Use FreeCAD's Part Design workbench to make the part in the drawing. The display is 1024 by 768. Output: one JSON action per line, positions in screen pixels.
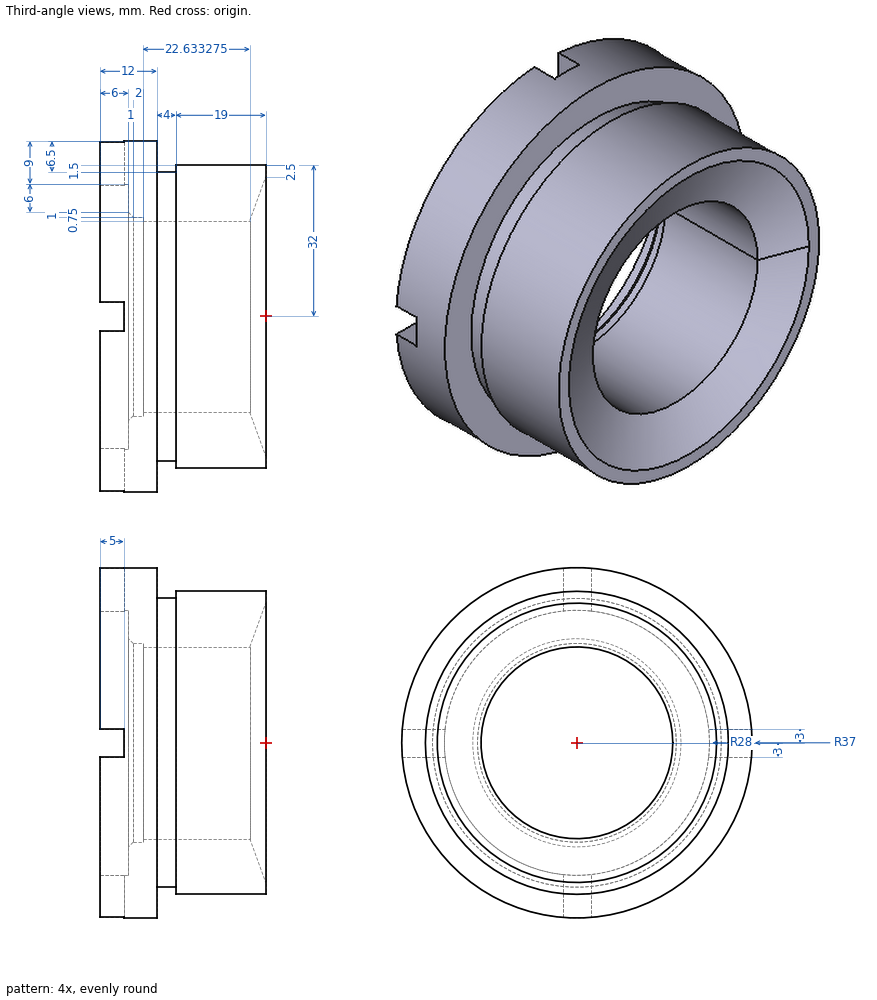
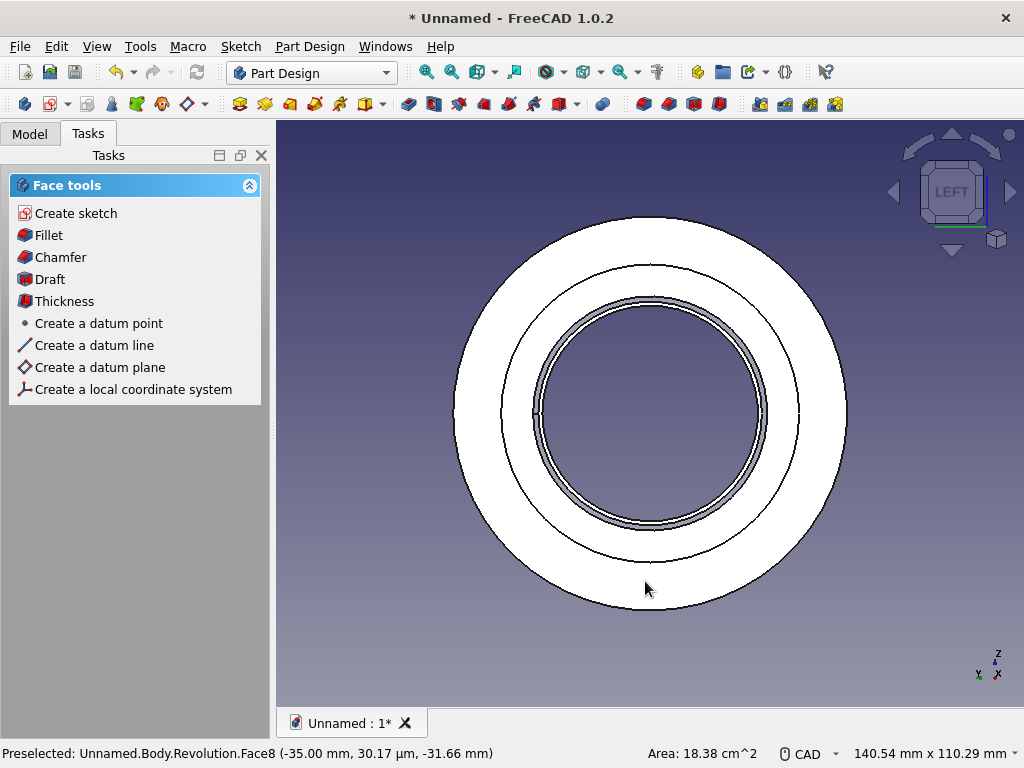
{"action": "left_click", "coordinate": [50, 104]}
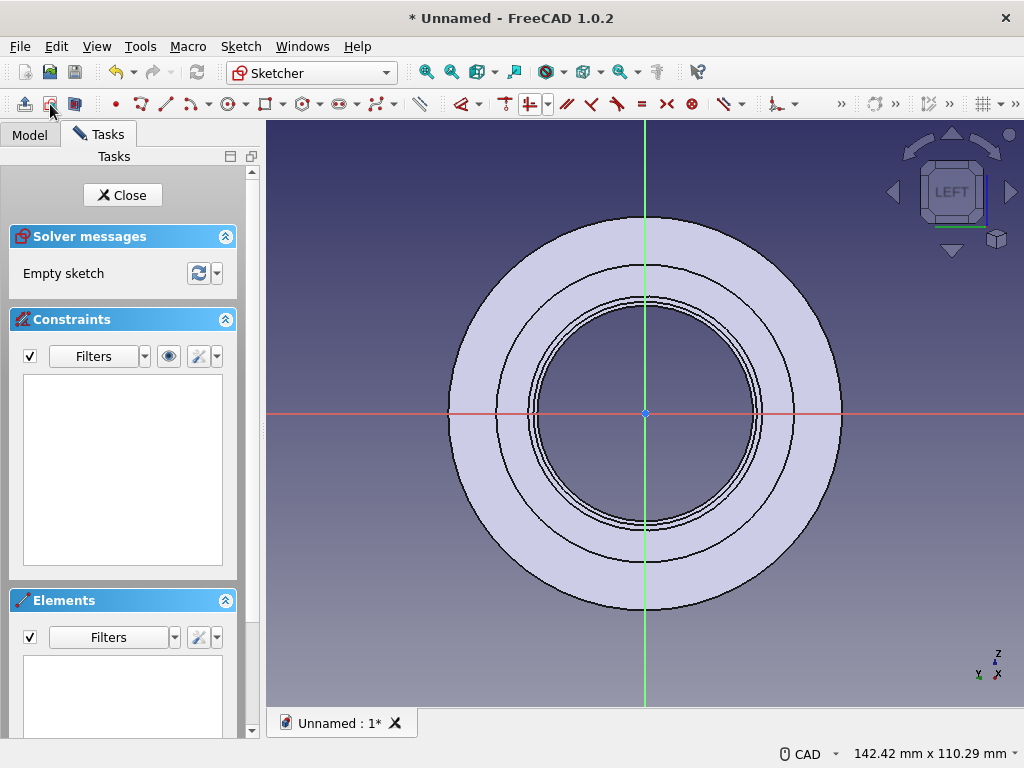
{"action": "scroll", "coordinate": [460, 414], "scroll_direction": "up", "scroll_amount": 11}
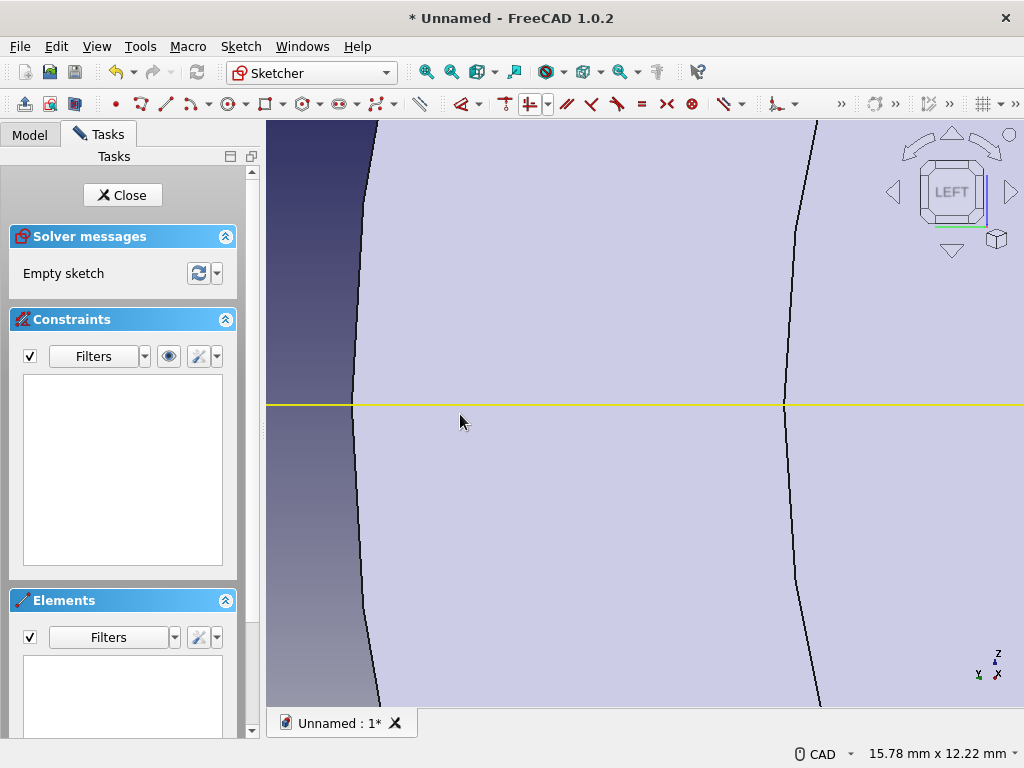
{"action": "left_click", "coordinate": [166, 104]}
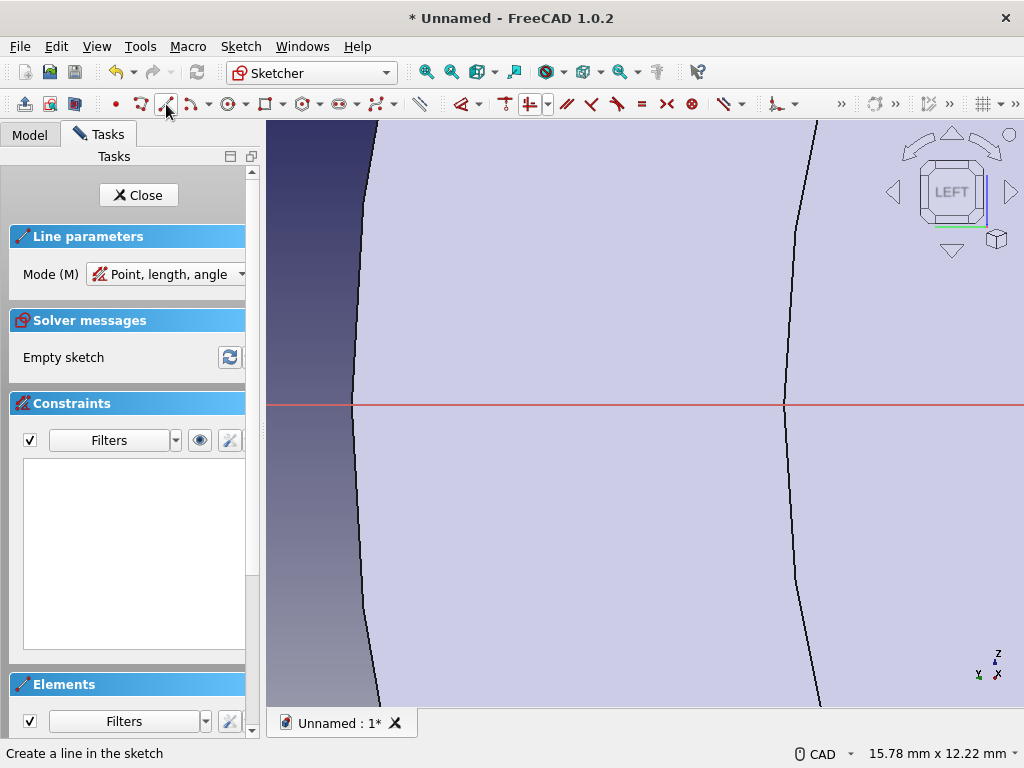
{"action": "left_click", "coordinate": [358, 550]}
{"action": "left_click", "coordinate": [792, 550]}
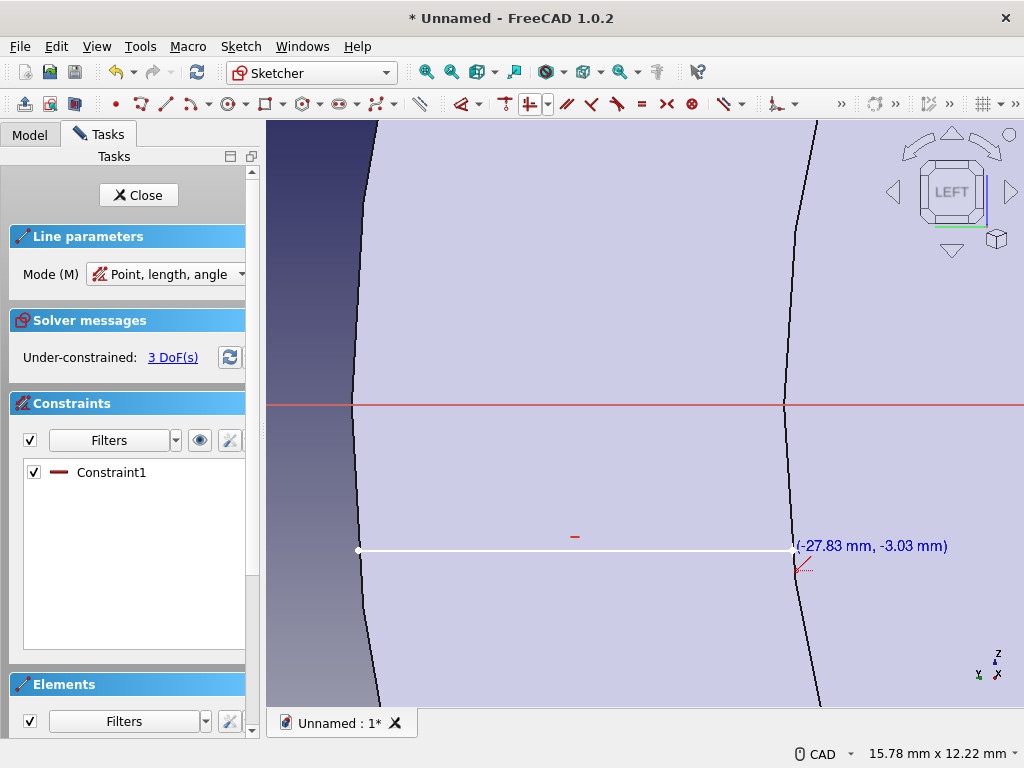
{"action": "left_click", "coordinate": [792, 261]}
{"action": "left_click", "coordinate": [358, 261]}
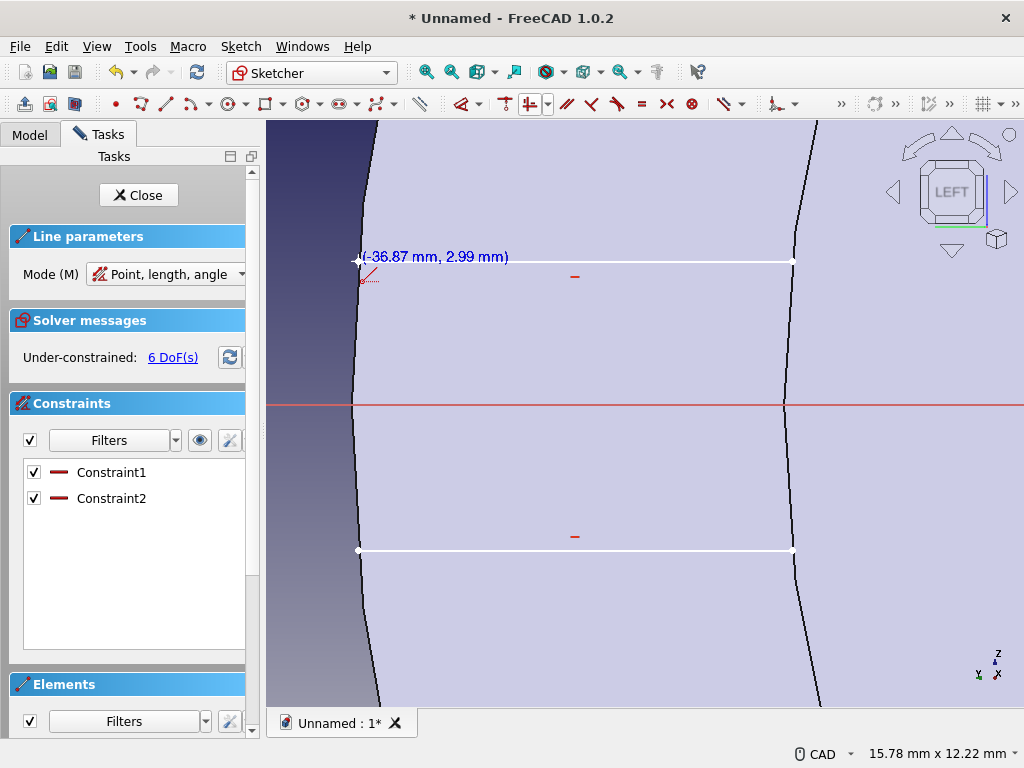
{"action": "left_click", "coordinate": [208, 104]}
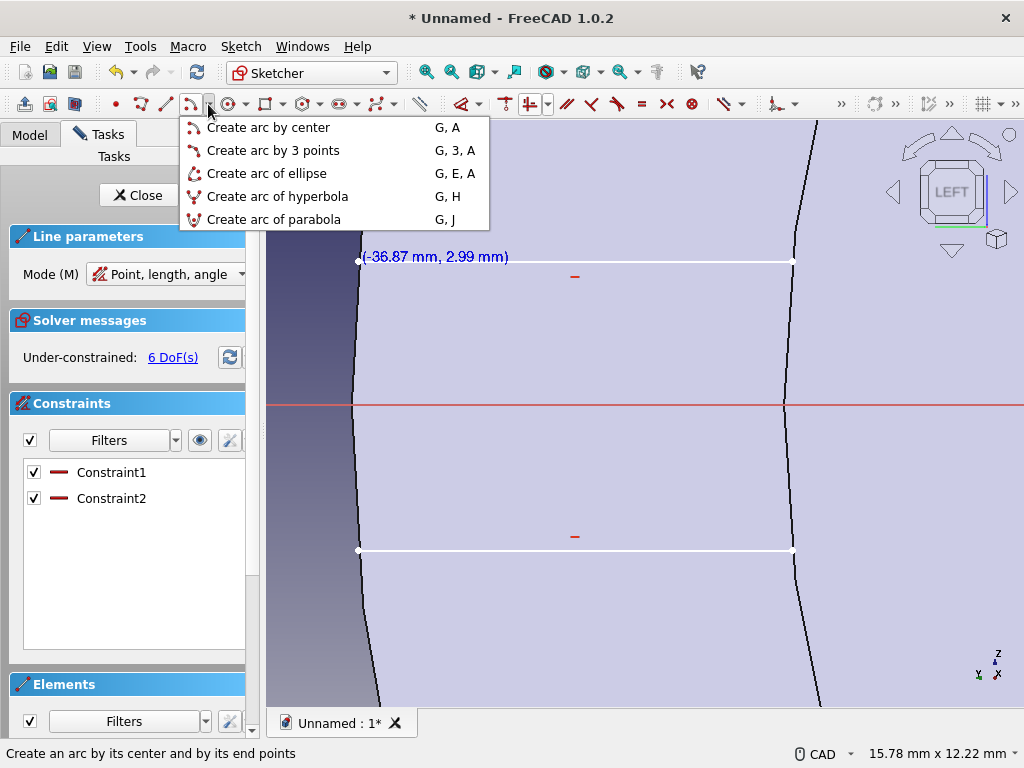
{"action": "left_click", "coordinate": [334, 150]}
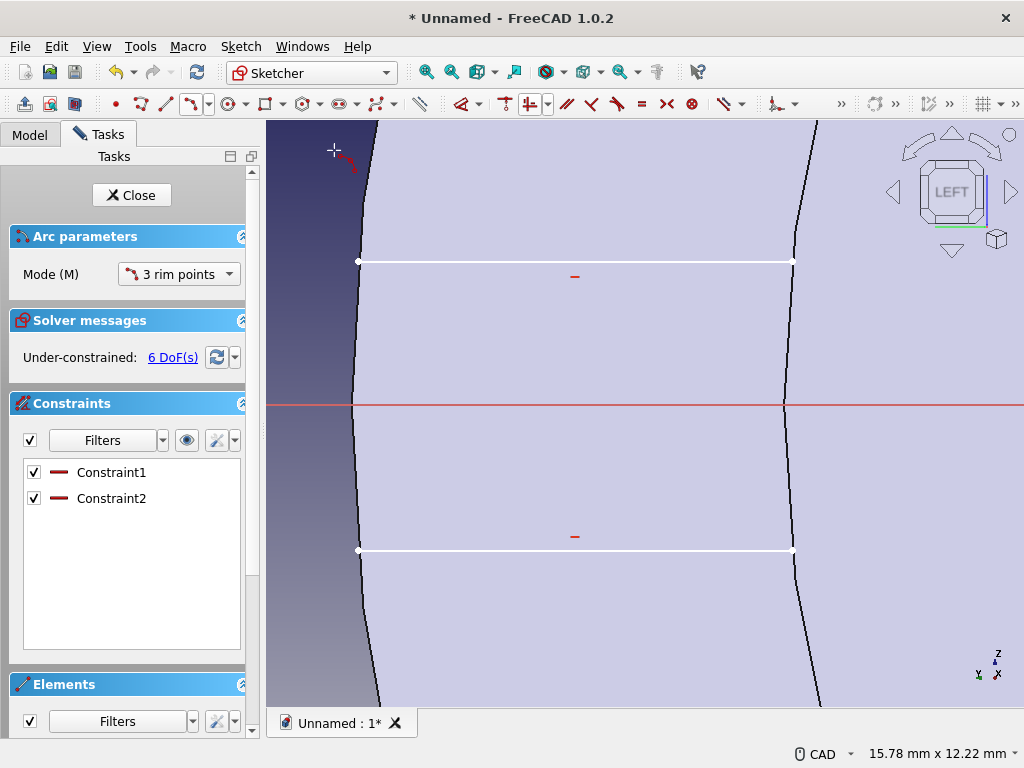
{"action": "left_click", "coordinate": [792, 551]}
{"action": "left_click", "coordinate": [792, 262]}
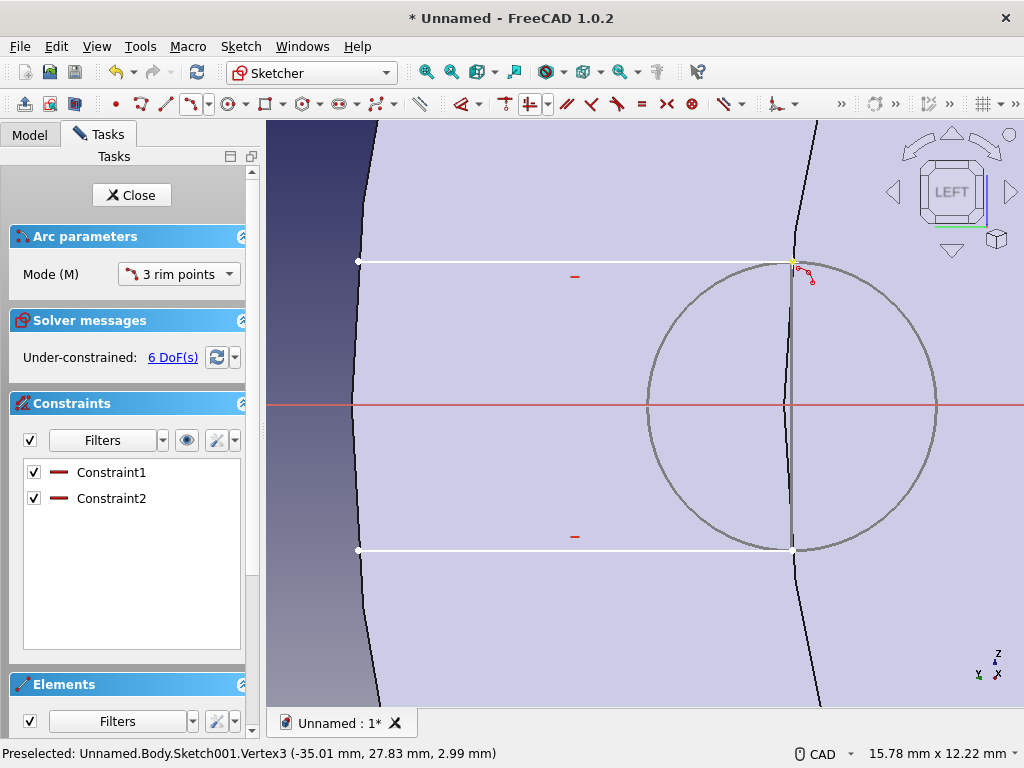
{"action": "scroll", "coordinate": [784, 377], "scroll_direction": "up", "scroll_amount": 4}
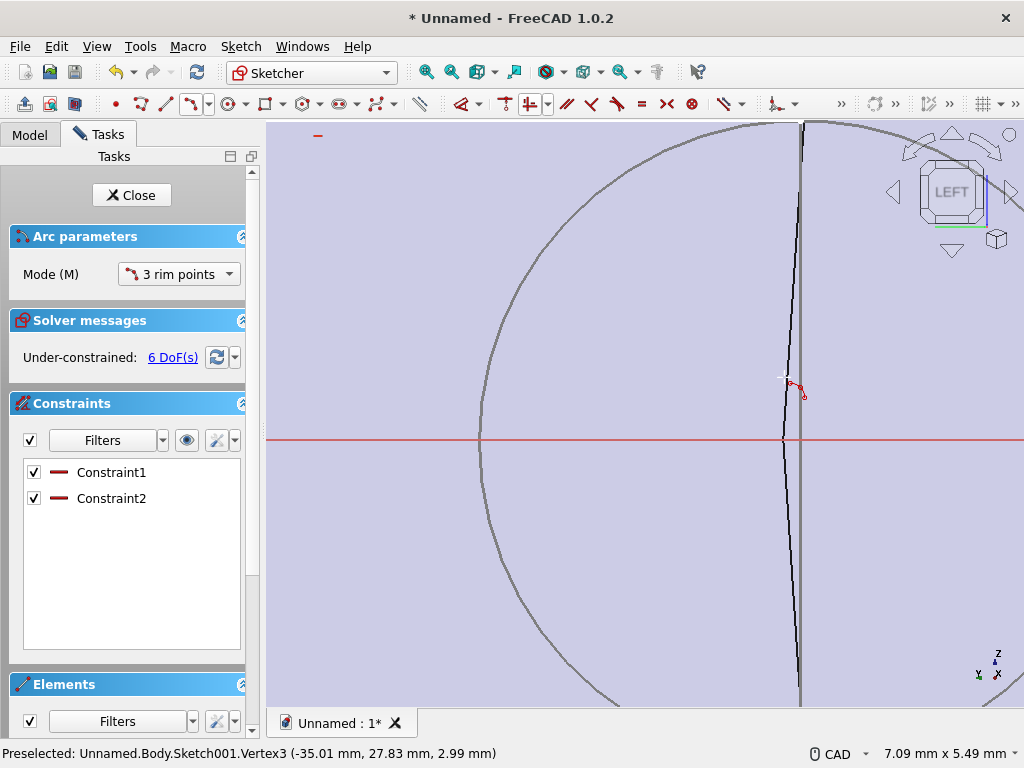
{"action": "left_click", "coordinate": [784, 376]}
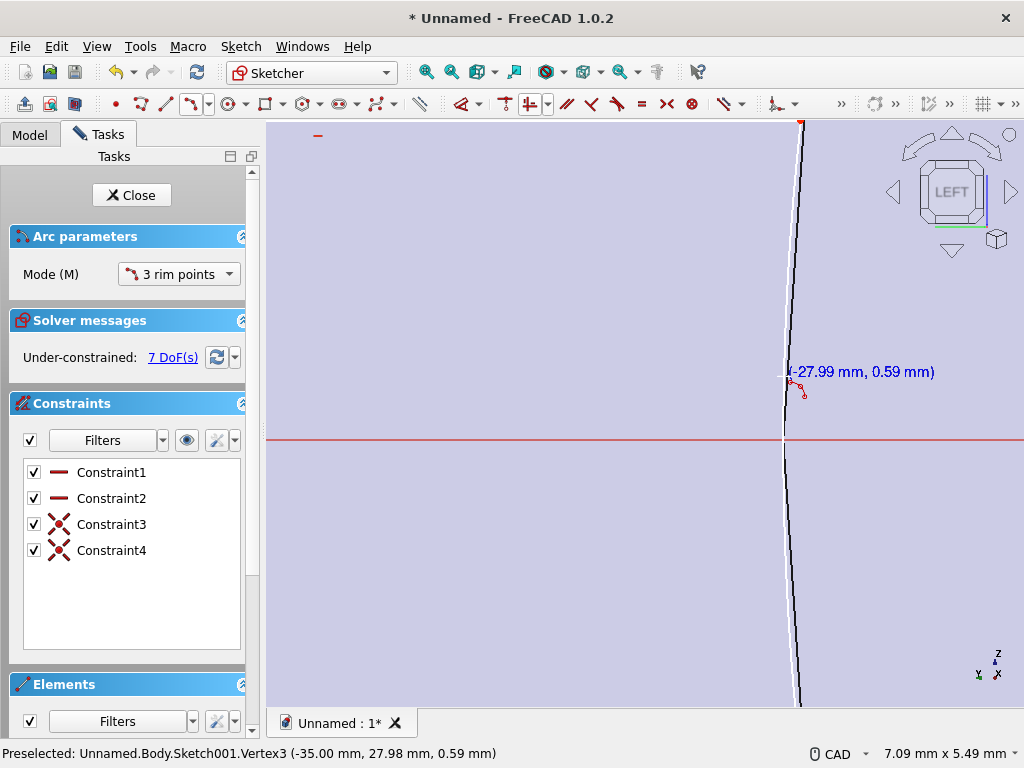
{"action": "scroll", "coordinate": [793, 392], "scroll_direction": "down", "scroll_amount": 4}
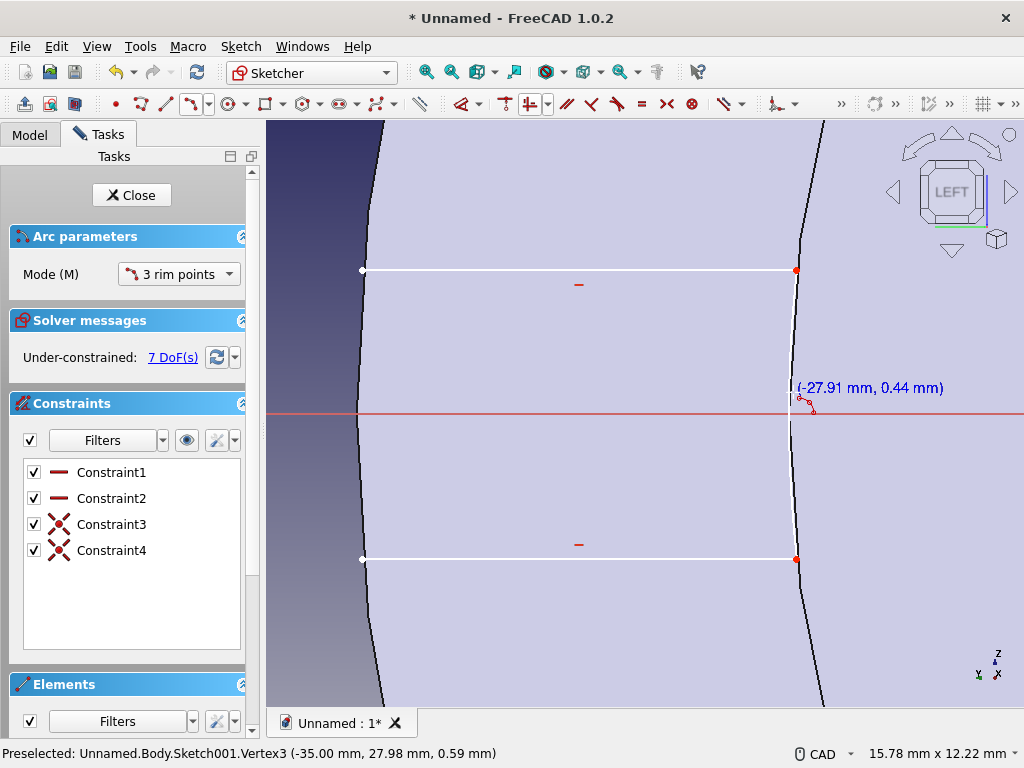
{"action": "left_click", "coordinate": [363, 270]}
{"action": "left_click", "coordinate": [363, 559]}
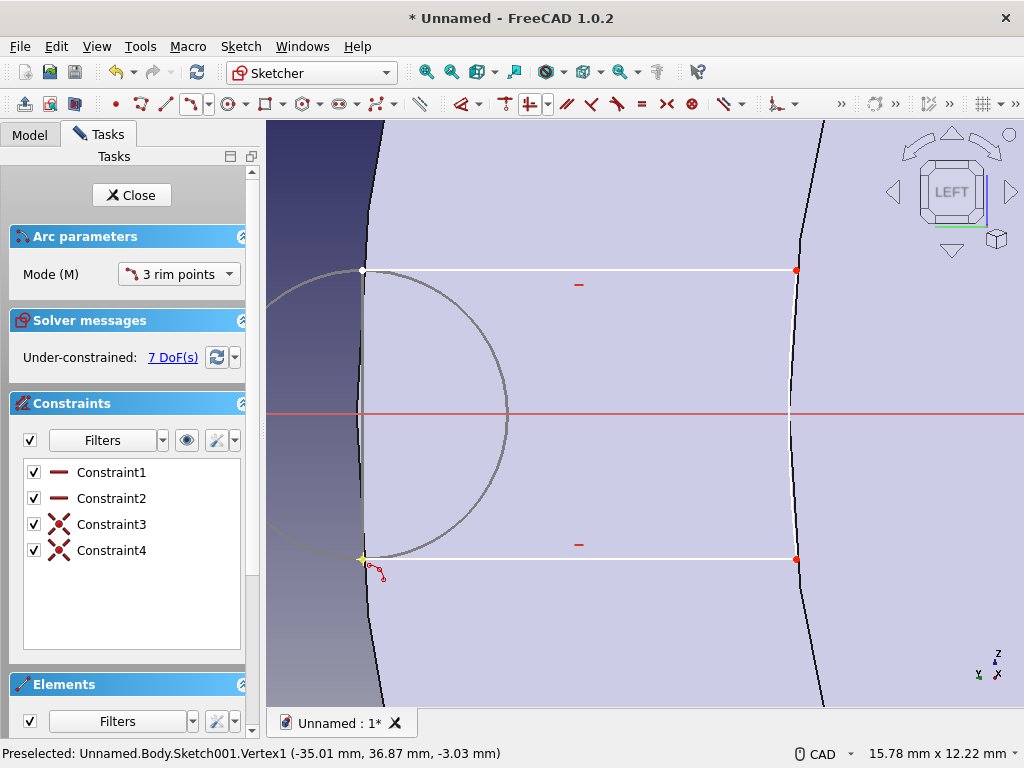
{"action": "scroll", "coordinate": [357, 385], "scroll_direction": "up", "scroll_amount": 6}